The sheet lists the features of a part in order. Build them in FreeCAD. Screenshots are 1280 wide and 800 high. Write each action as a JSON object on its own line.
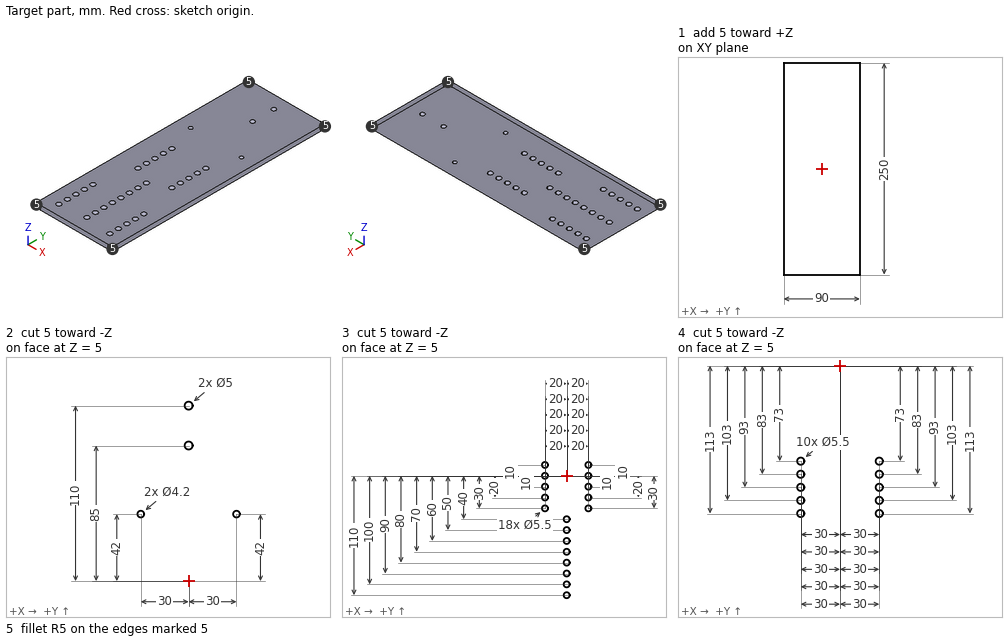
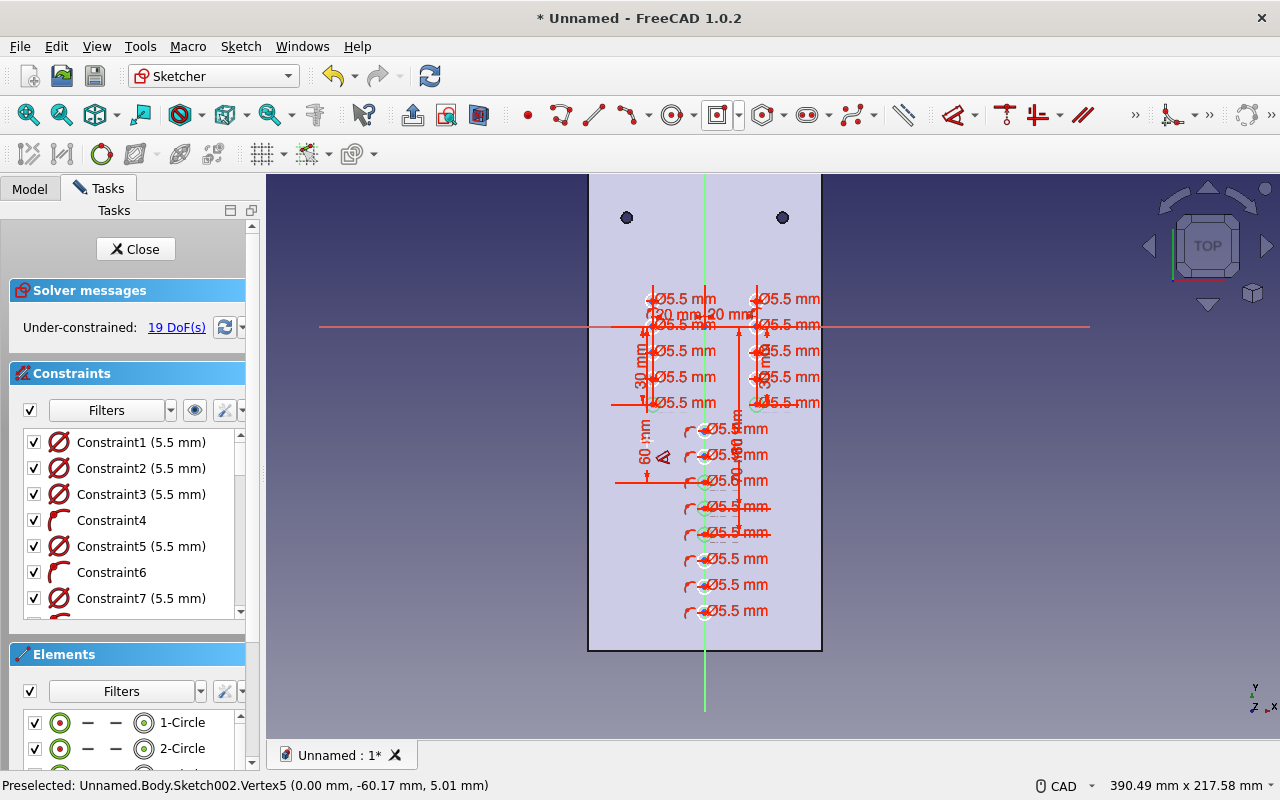
{"action": "left_click", "coordinate": [705, 457]}
{"action": "left_click", "coordinate": [739, 392]}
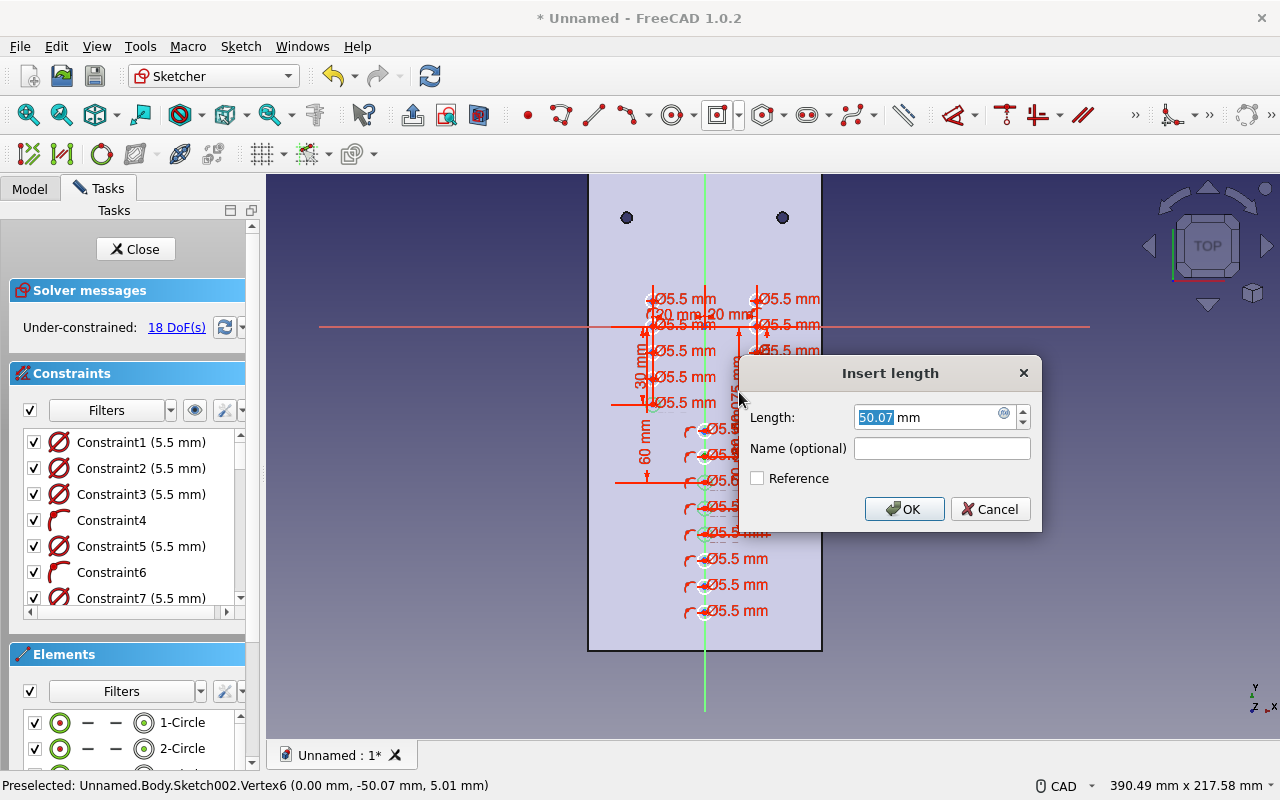
{"action": "type", "text": "50"}
{"action": "key", "text": "Return"}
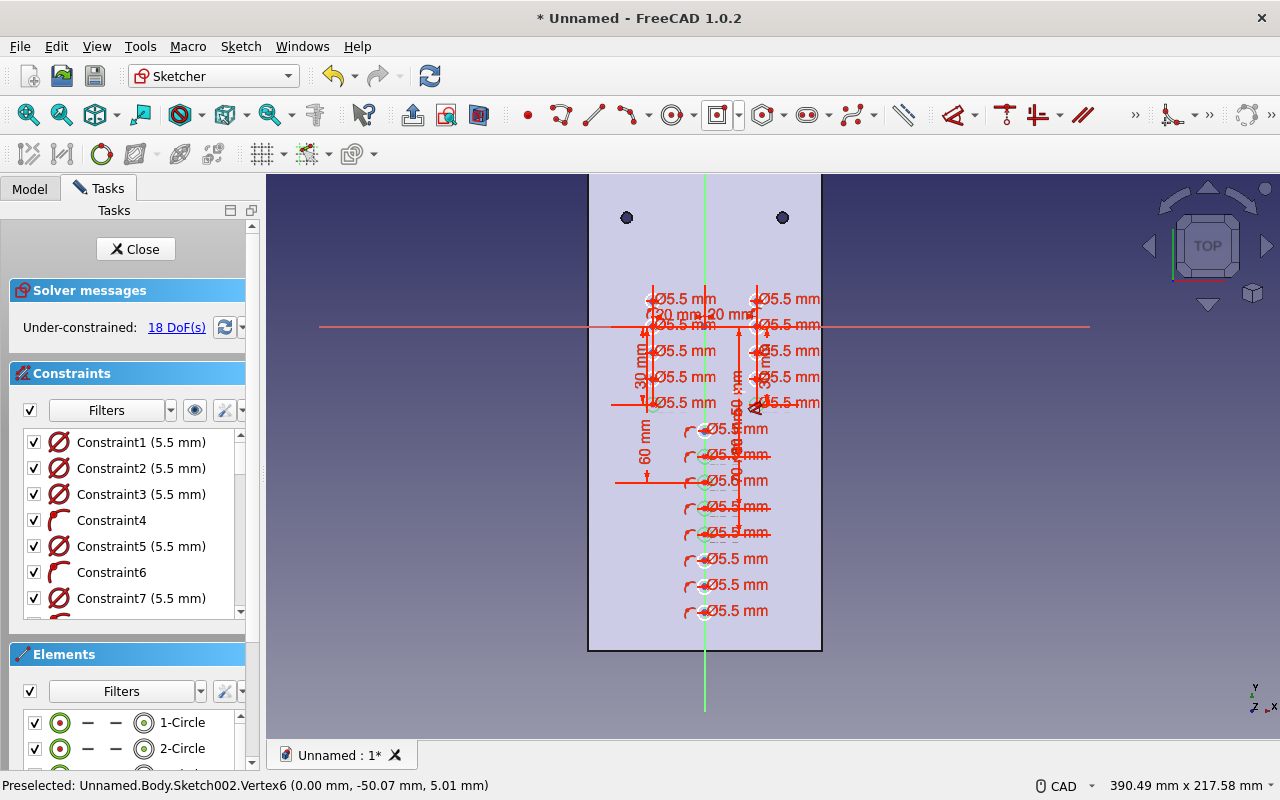
{"action": "left_click", "coordinate": [705, 431]}
{"action": "left_click", "coordinate": [739, 342]}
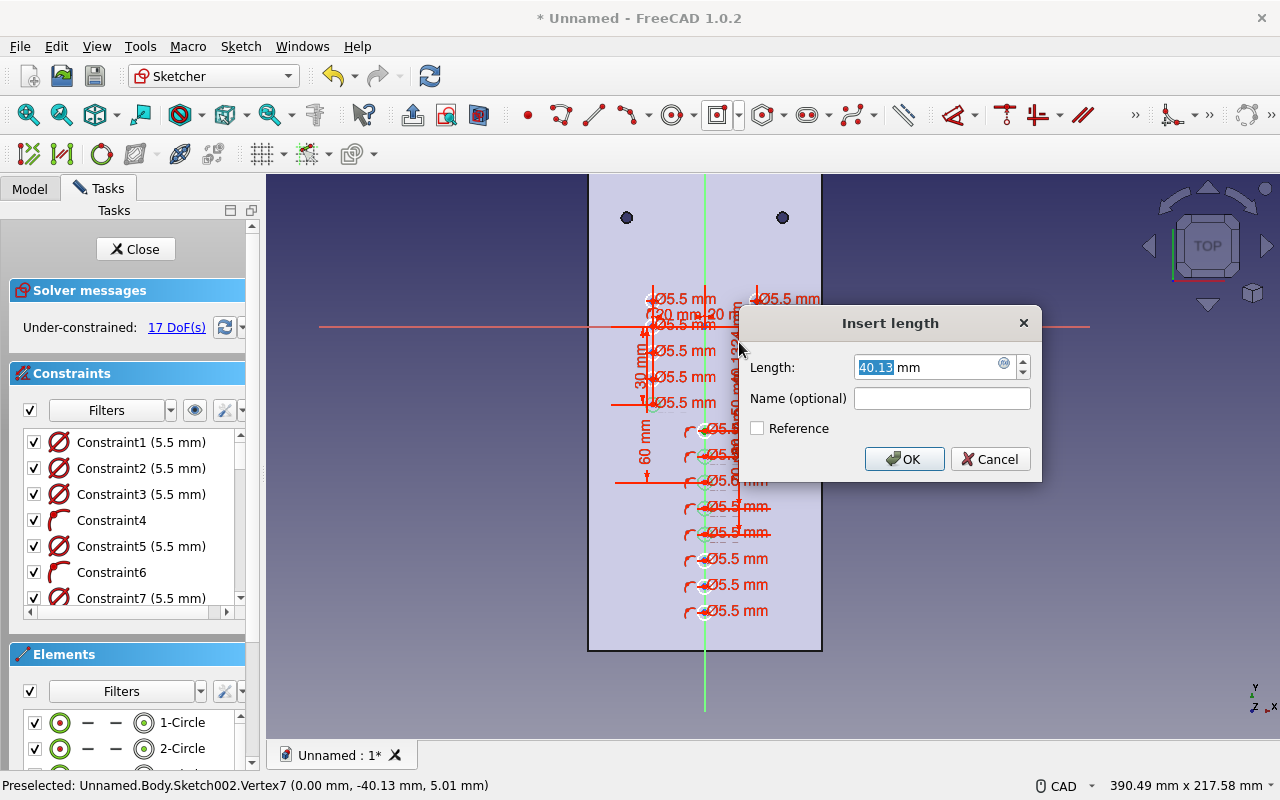
{"action": "type", "text": "40"}
{"action": "key", "text": "Return"}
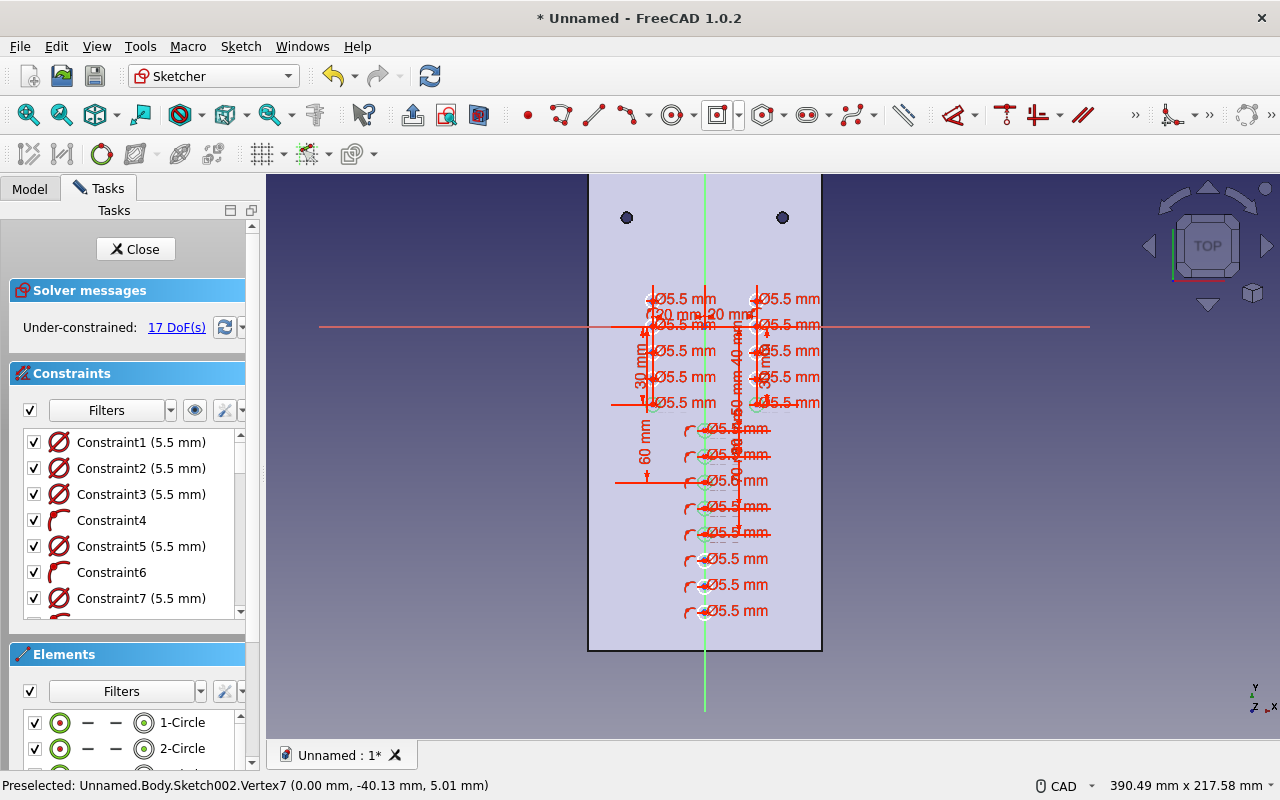
{"action": "left_click", "coordinate": [705, 561]}
{"action": "left_click", "coordinate": [739, 498]}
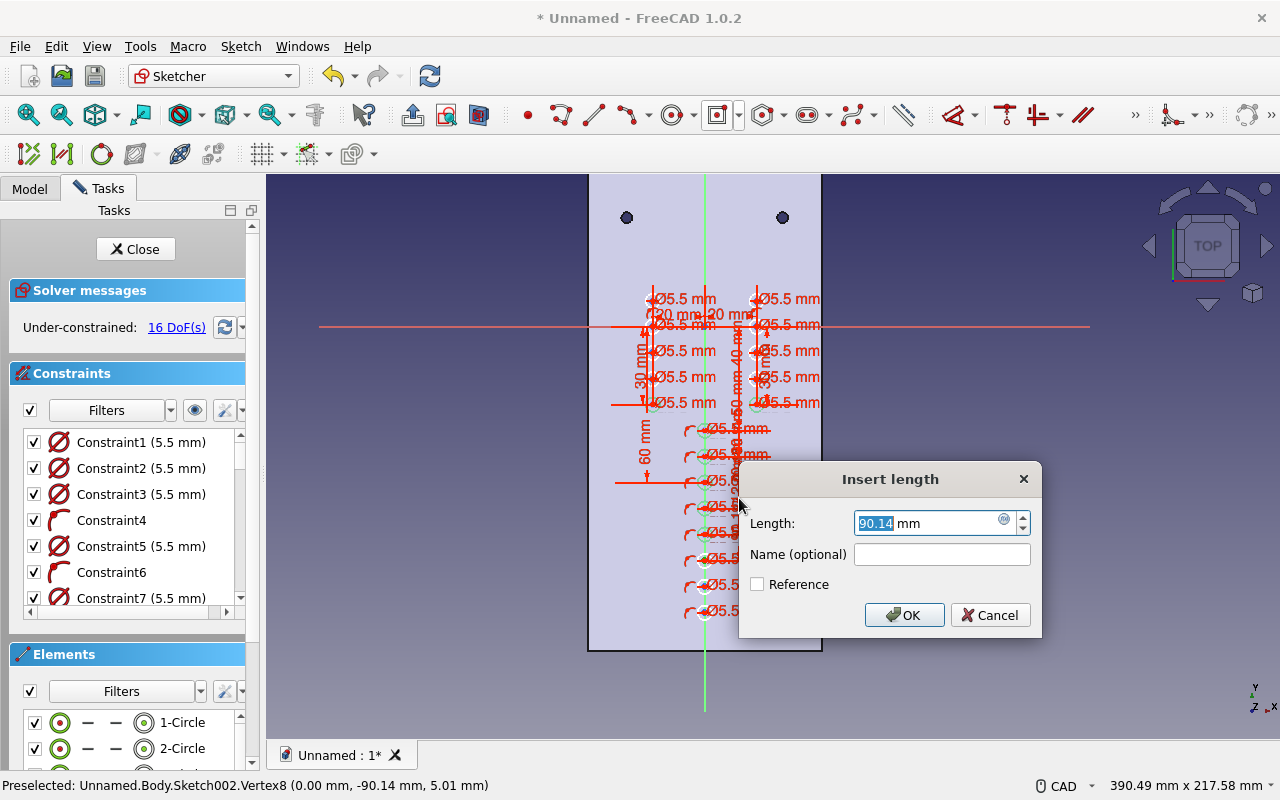
{"action": "type", "text": "90"}
{"action": "key", "text": "Return"}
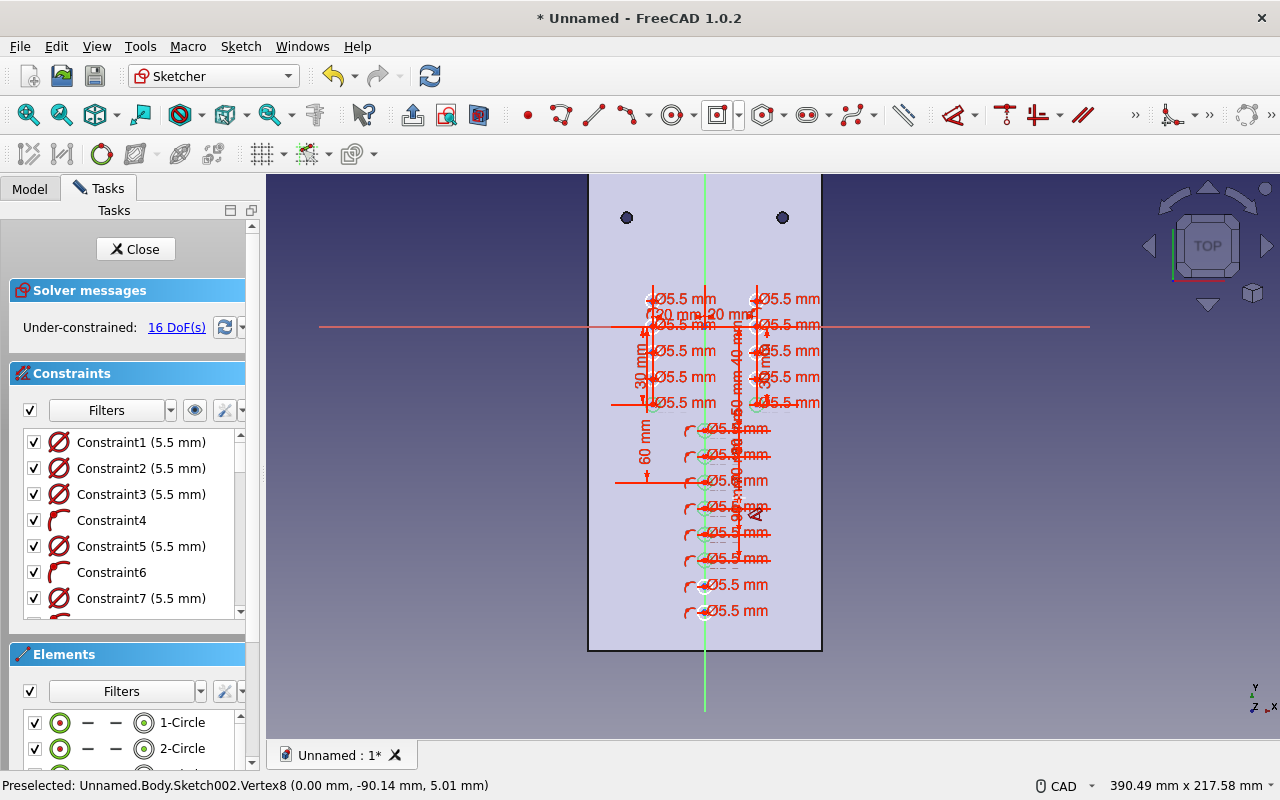
{"action": "left_click", "coordinate": [653, 379]}
{"action": "left_click", "coordinate": [679, 293]}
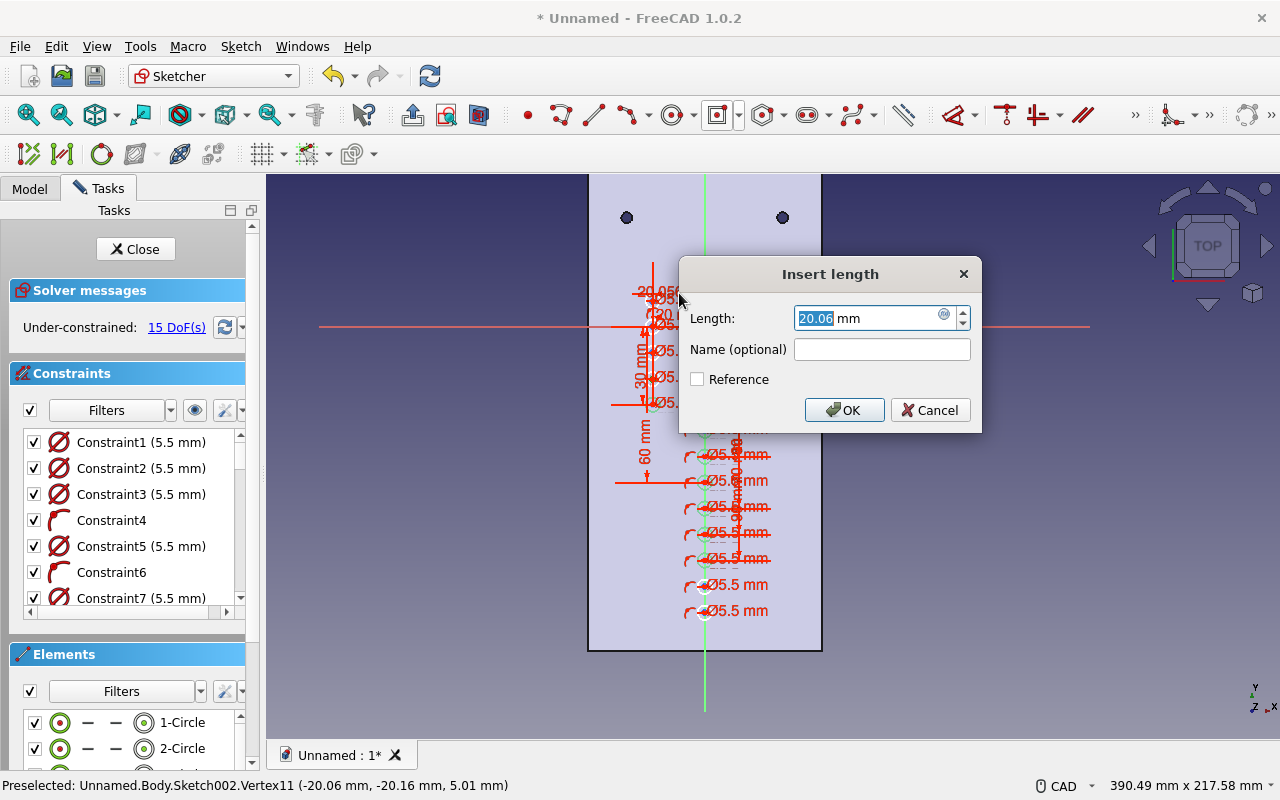
{"action": "type", "text": "20"}
{"action": "key", "text": "Return"}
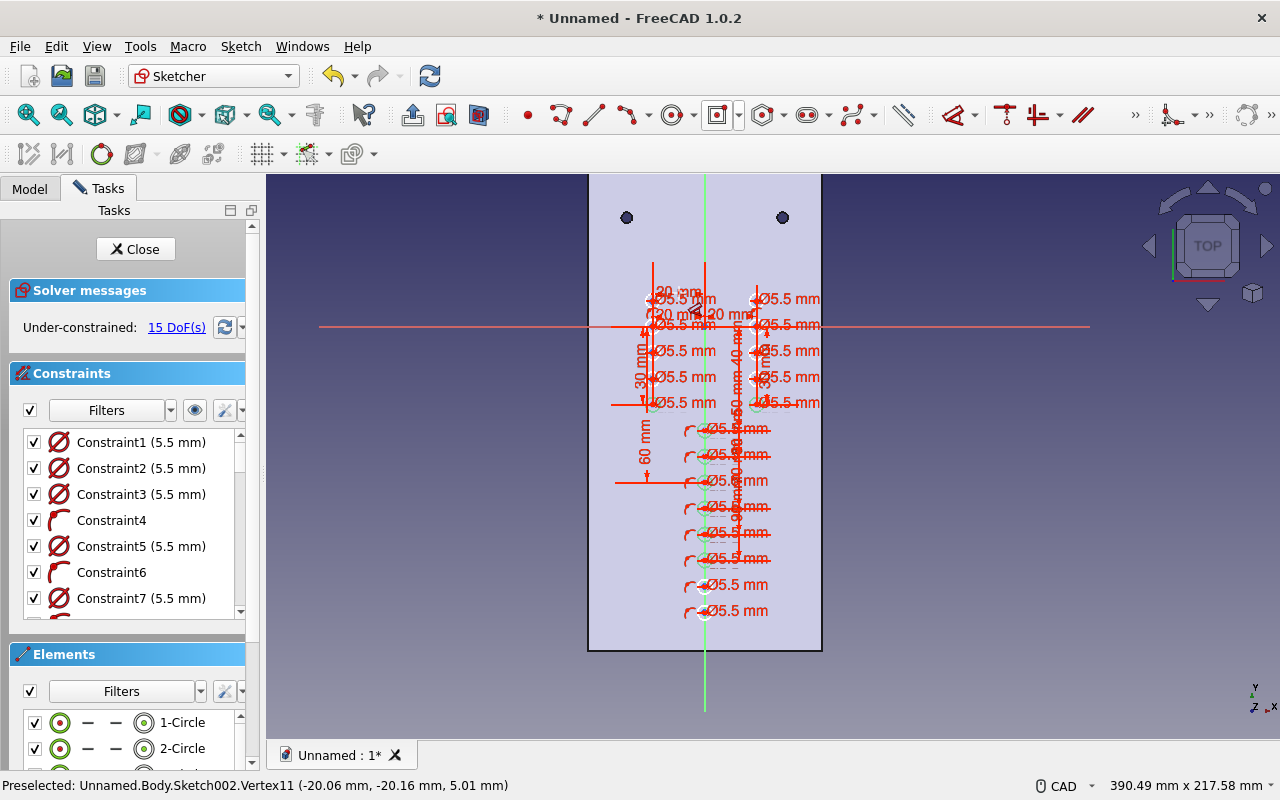
{"action": "left_click", "coordinate": [653, 379]}
{"action": "left_click", "coordinate": [619, 341]}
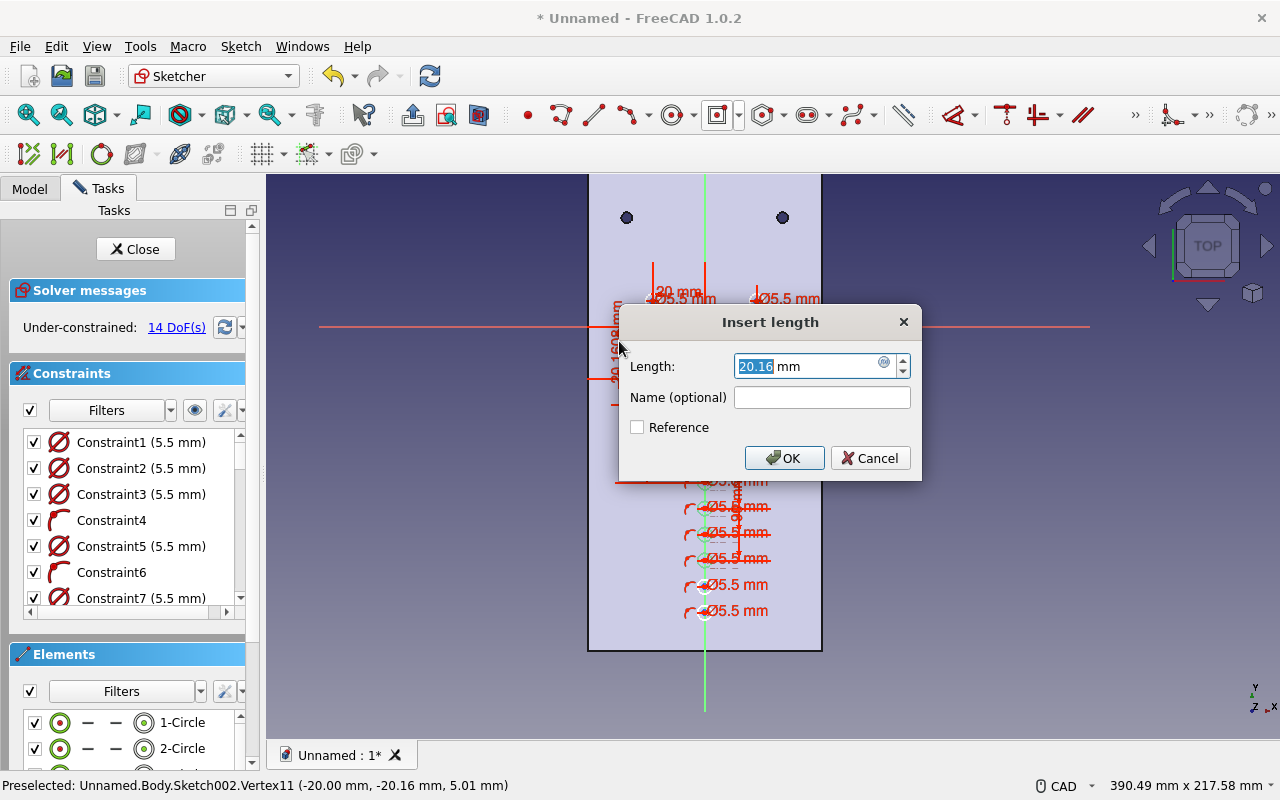
{"action": "type", "text": "20"}
{"action": "key", "text": "Return"}